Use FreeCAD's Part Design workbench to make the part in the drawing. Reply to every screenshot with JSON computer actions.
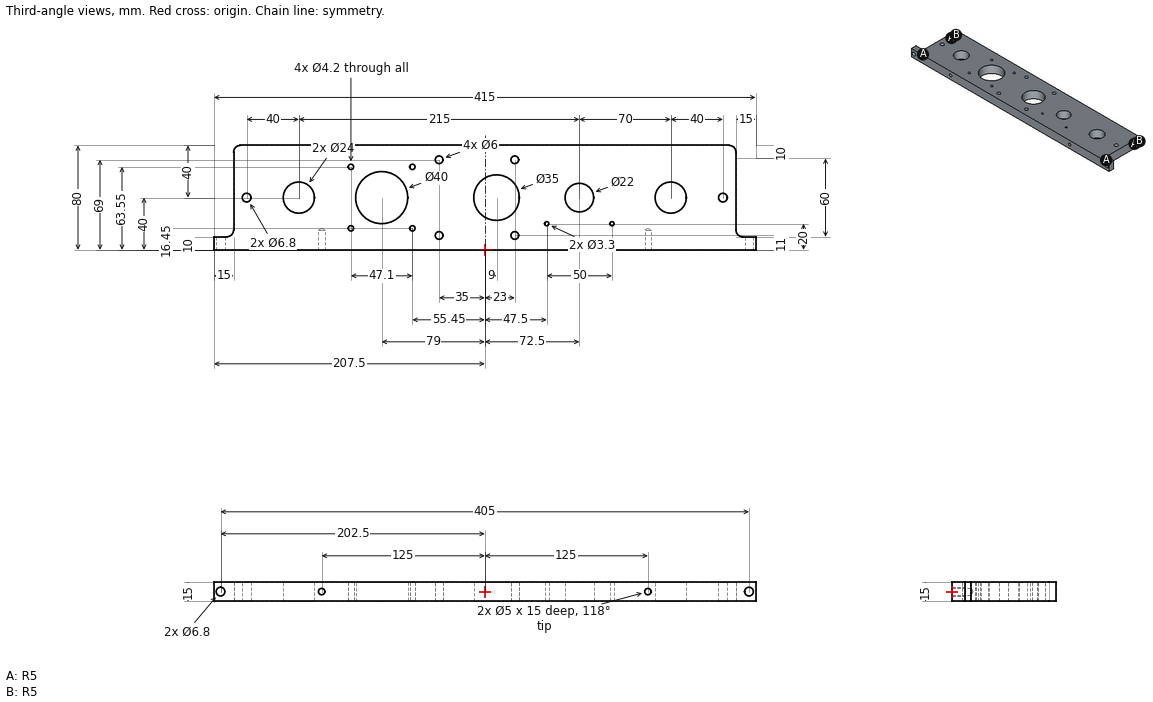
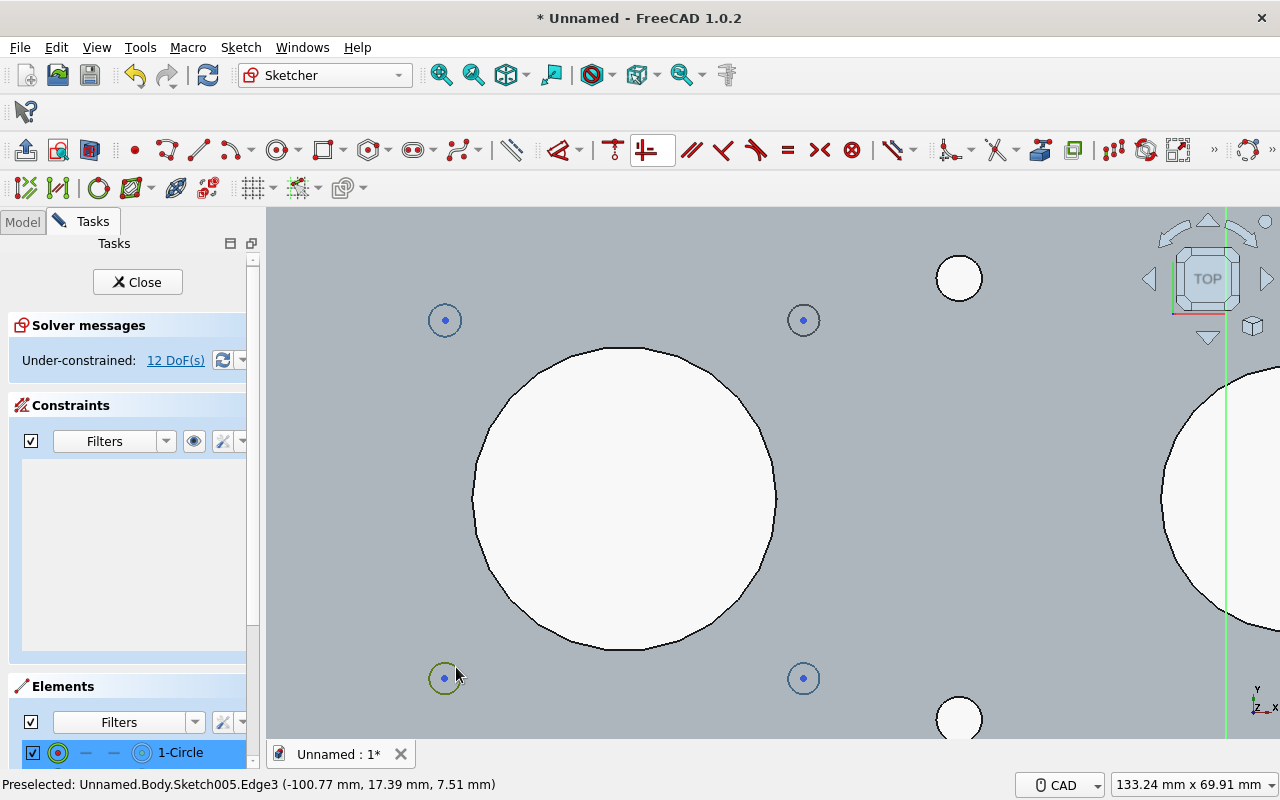
{"action": "left_click", "coordinate": [815, 309]}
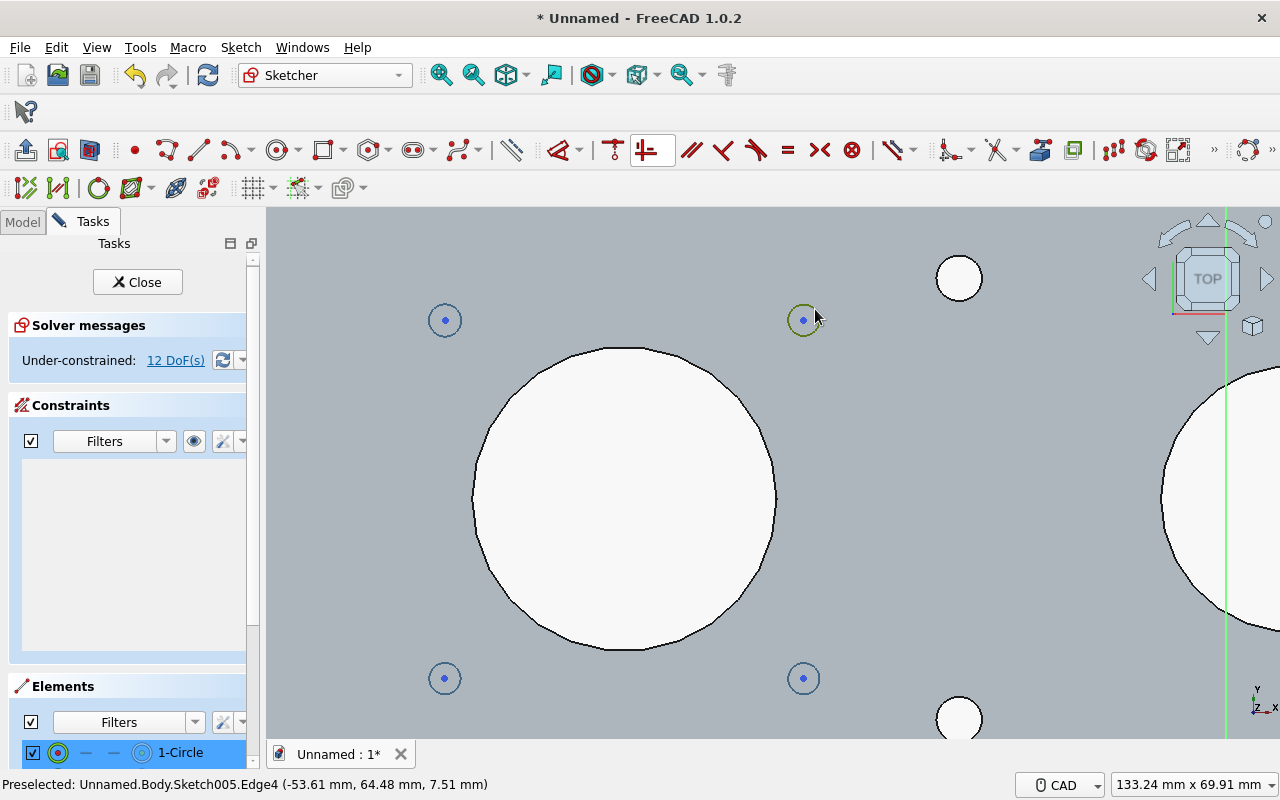
{"action": "left_click", "coordinate": [788, 150]}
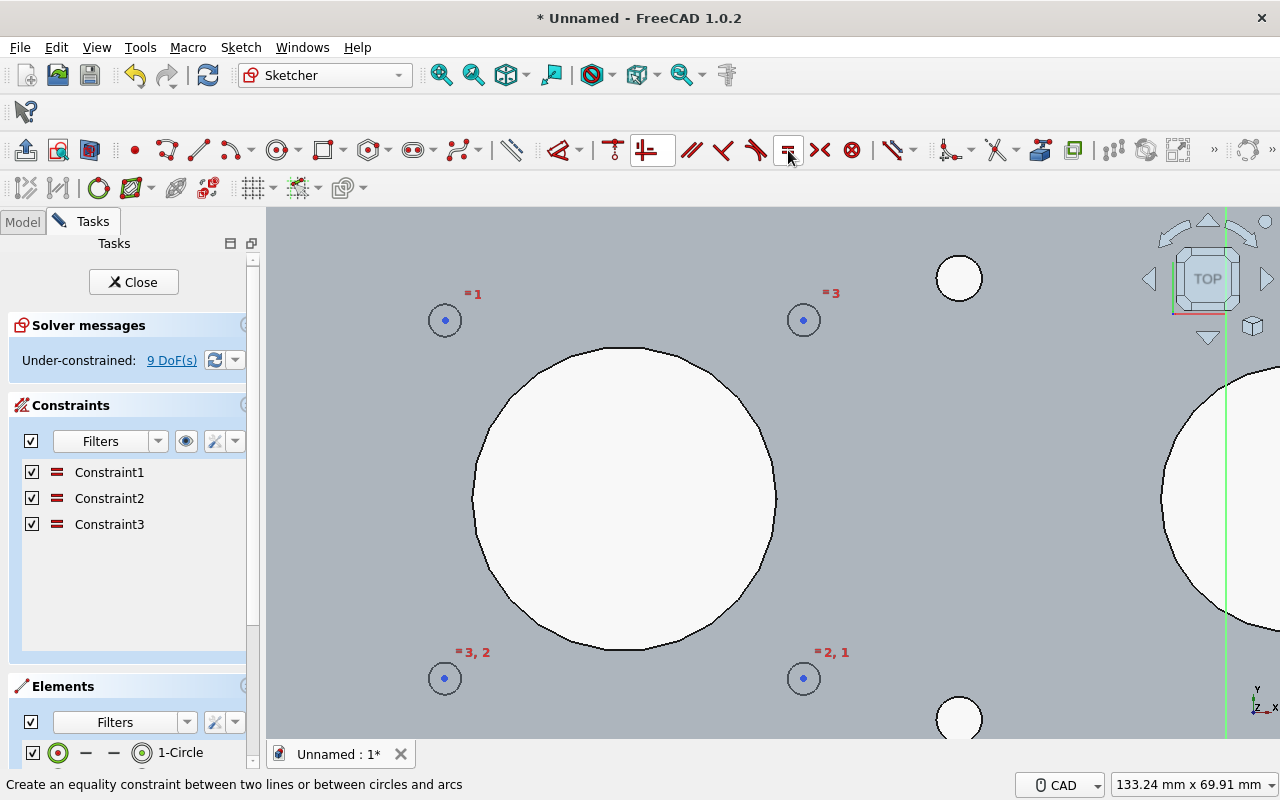
{"action": "left_click", "coordinate": [445, 320]}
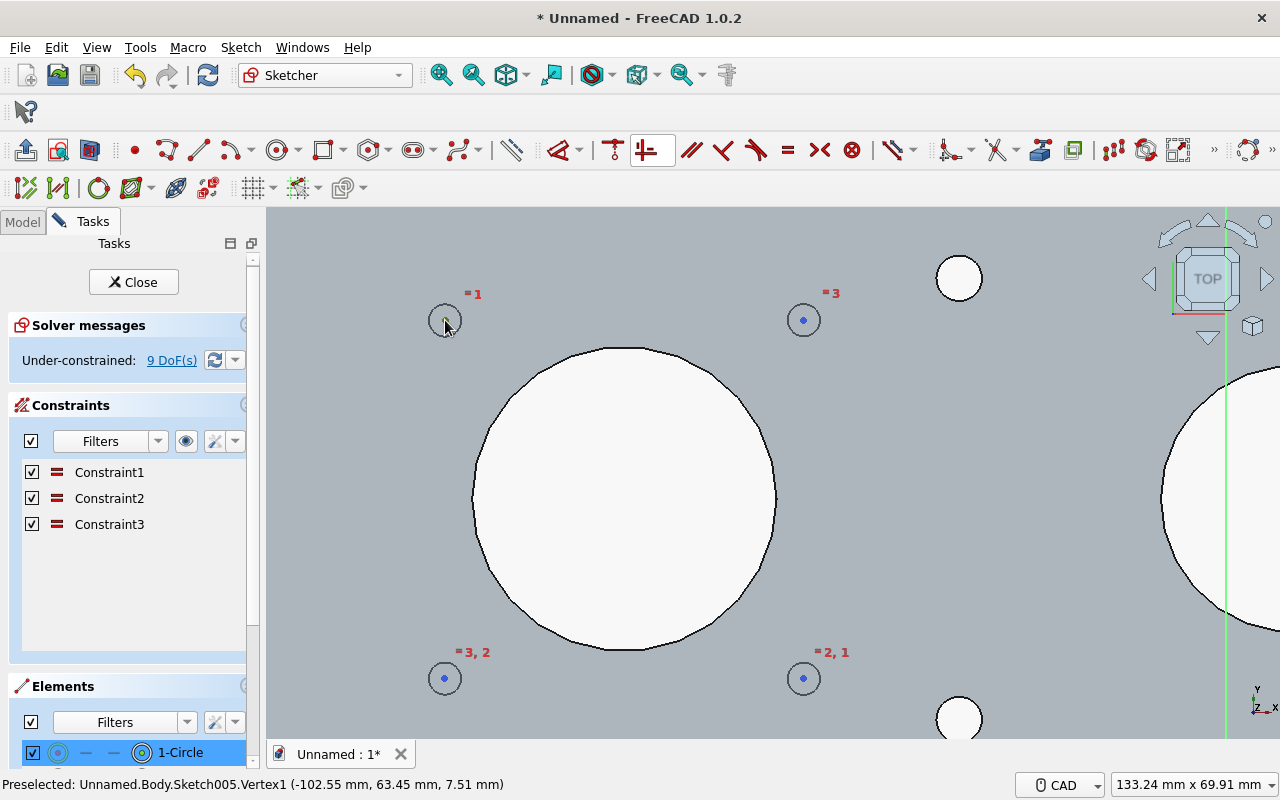
{"action": "left_click", "coordinate": [445, 679]}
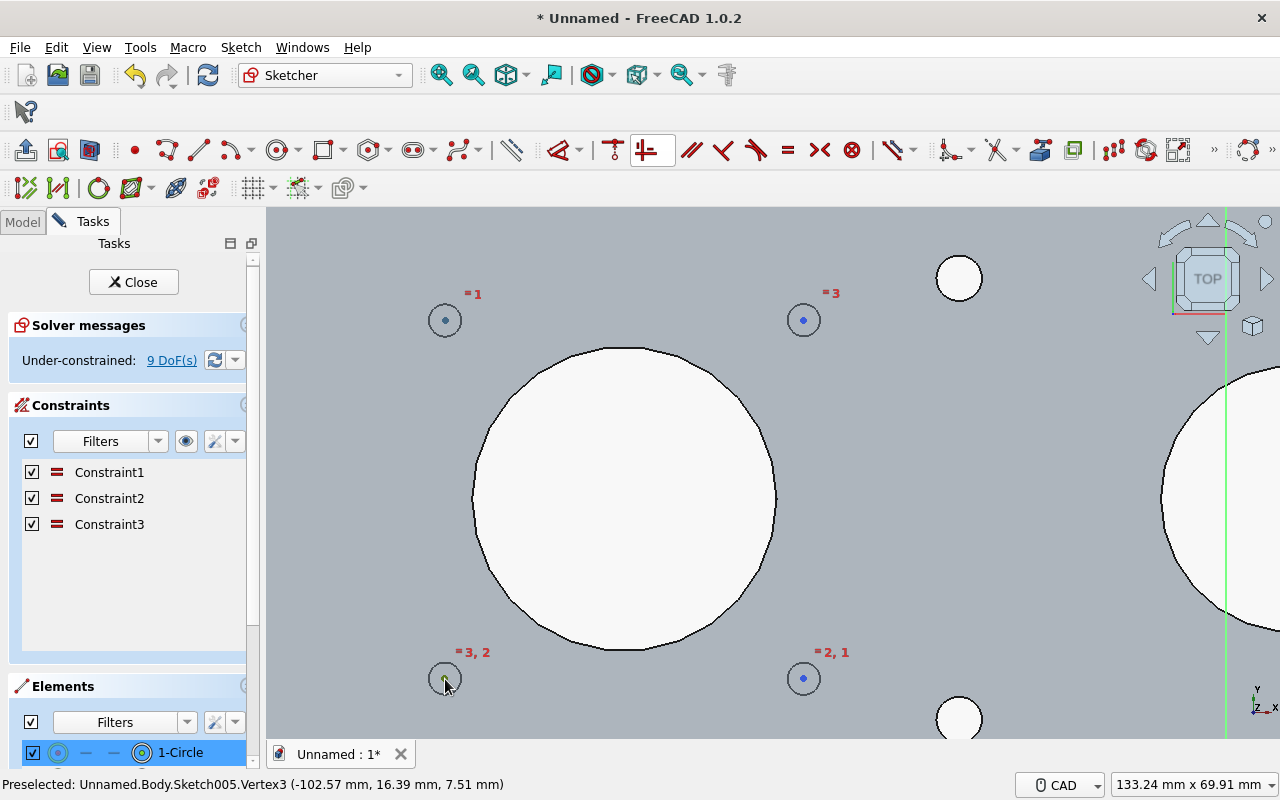
{"action": "key", "text": "v"}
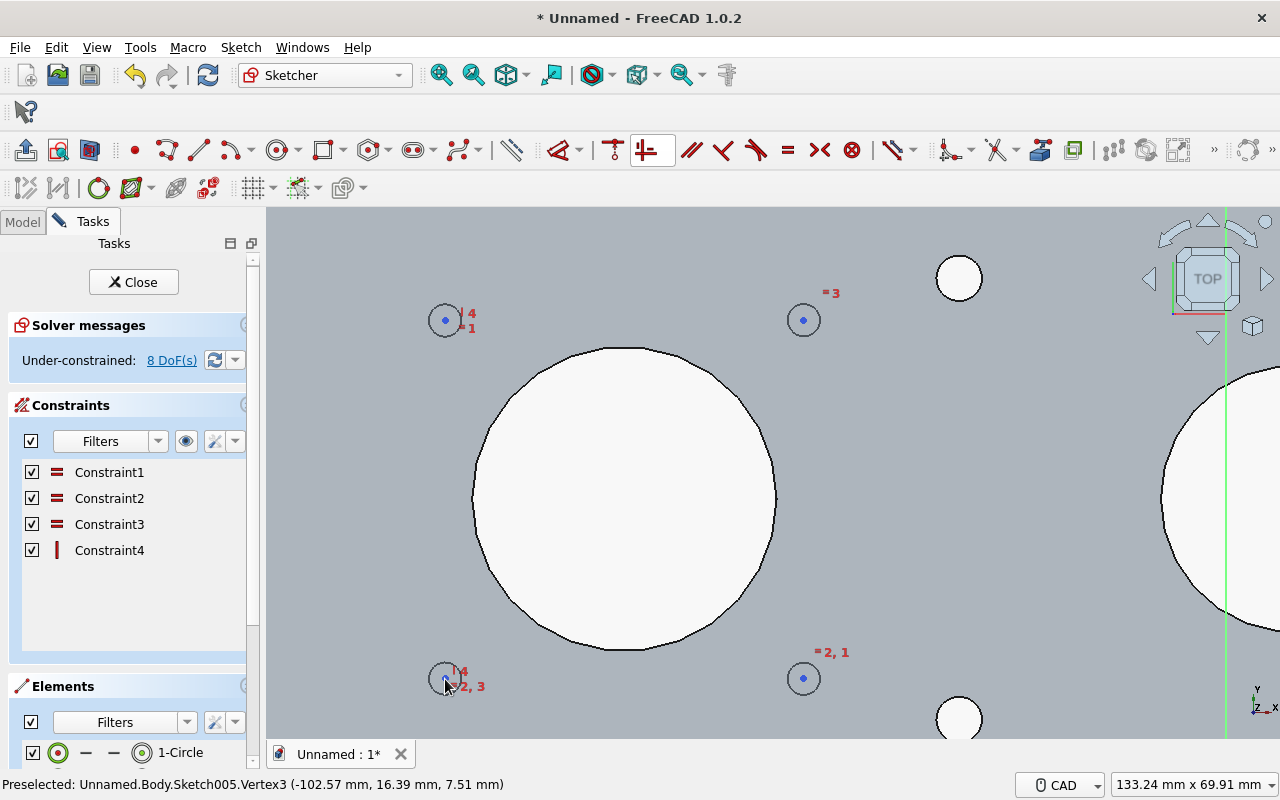
{"action": "left_click", "coordinate": [804, 679]}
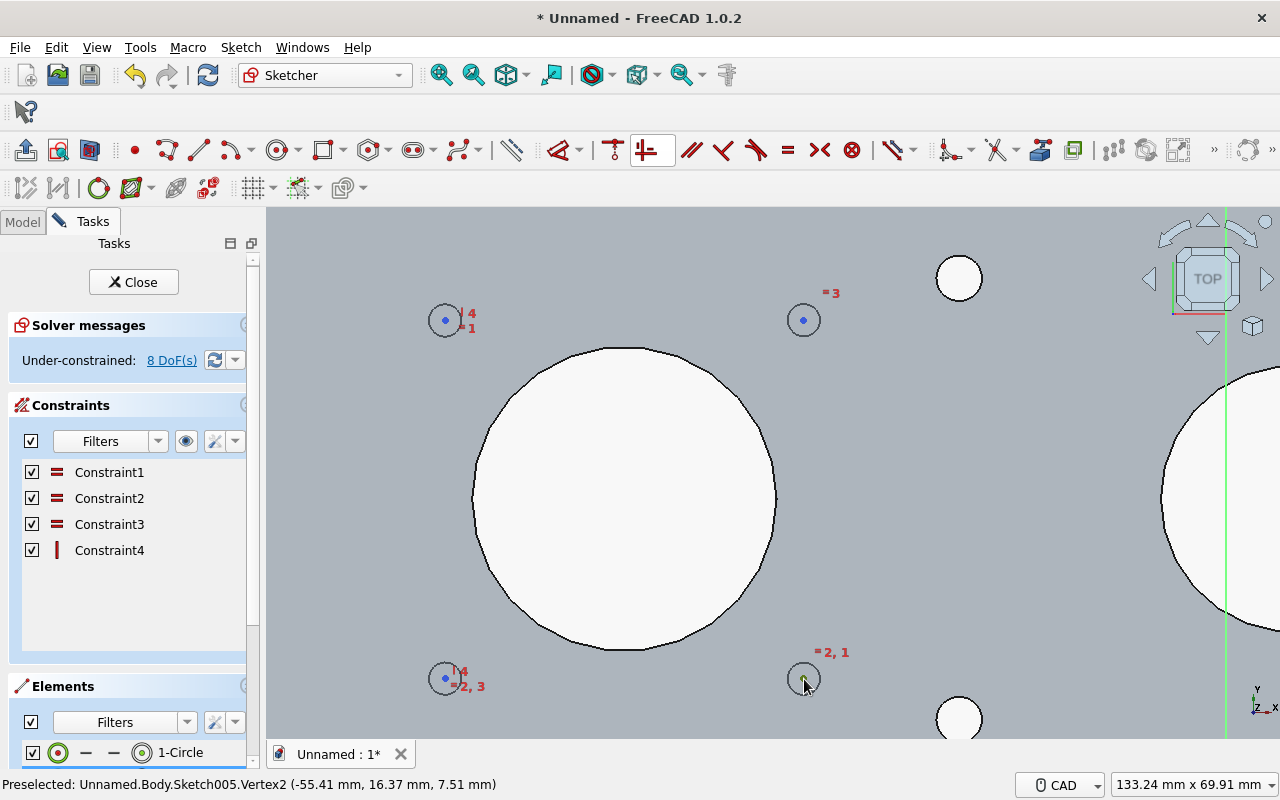
{"action": "left_click", "coordinate": [445, 679]}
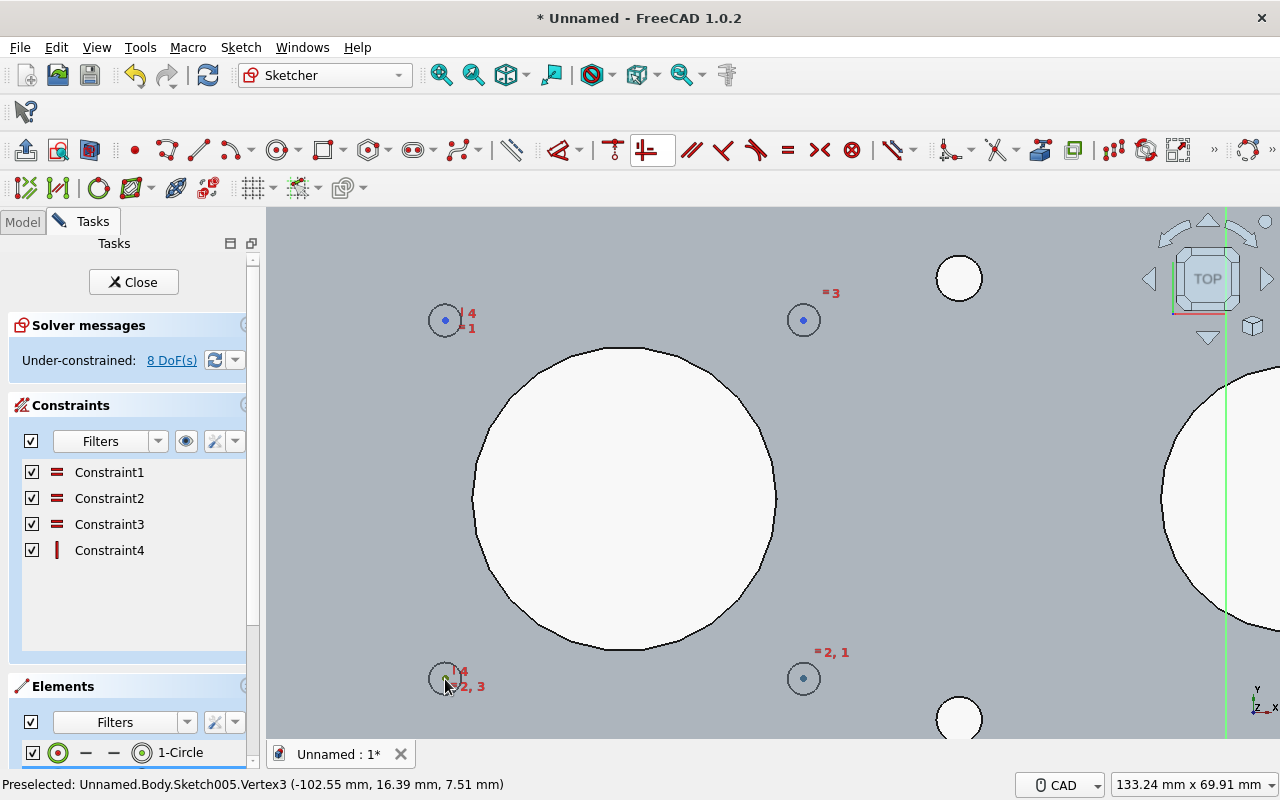
{"action": "left_click", "coordinate": [670, 150]}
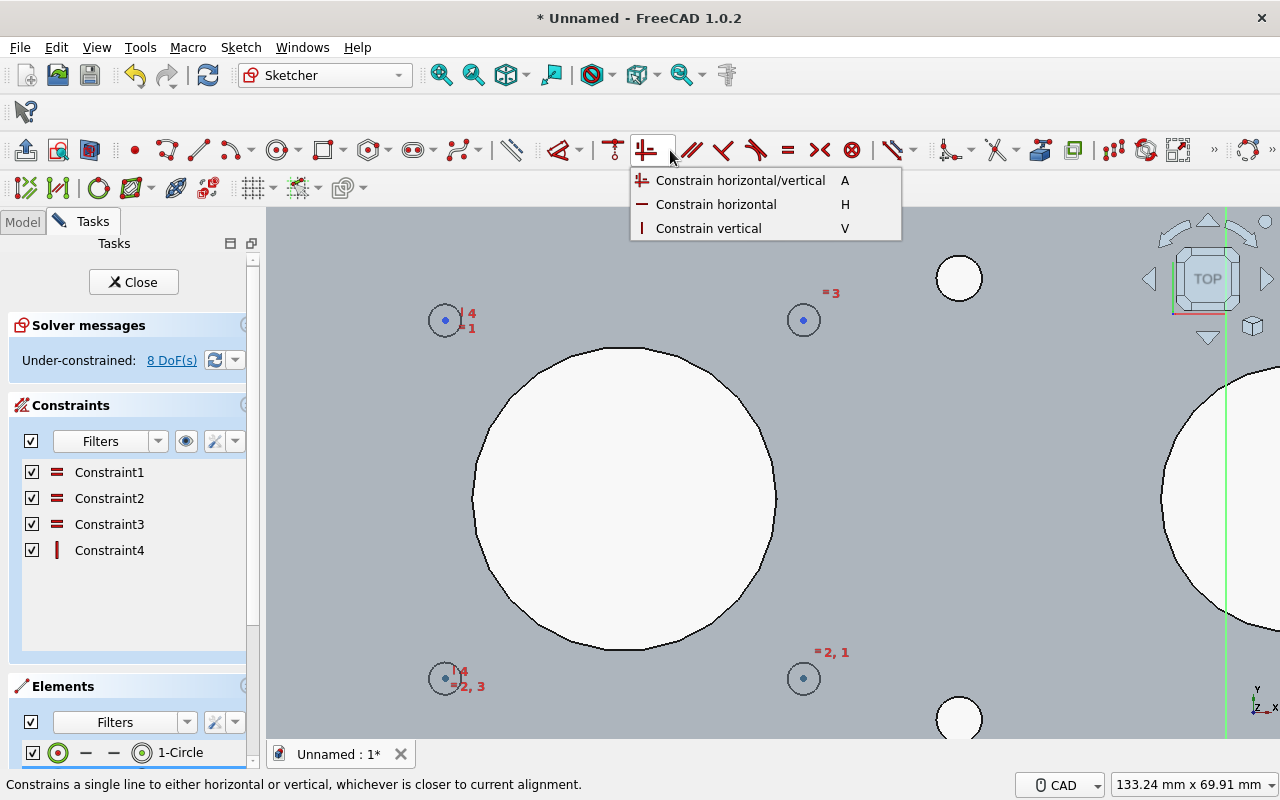
{"action": "left_click", "coordinate": [766, 204]}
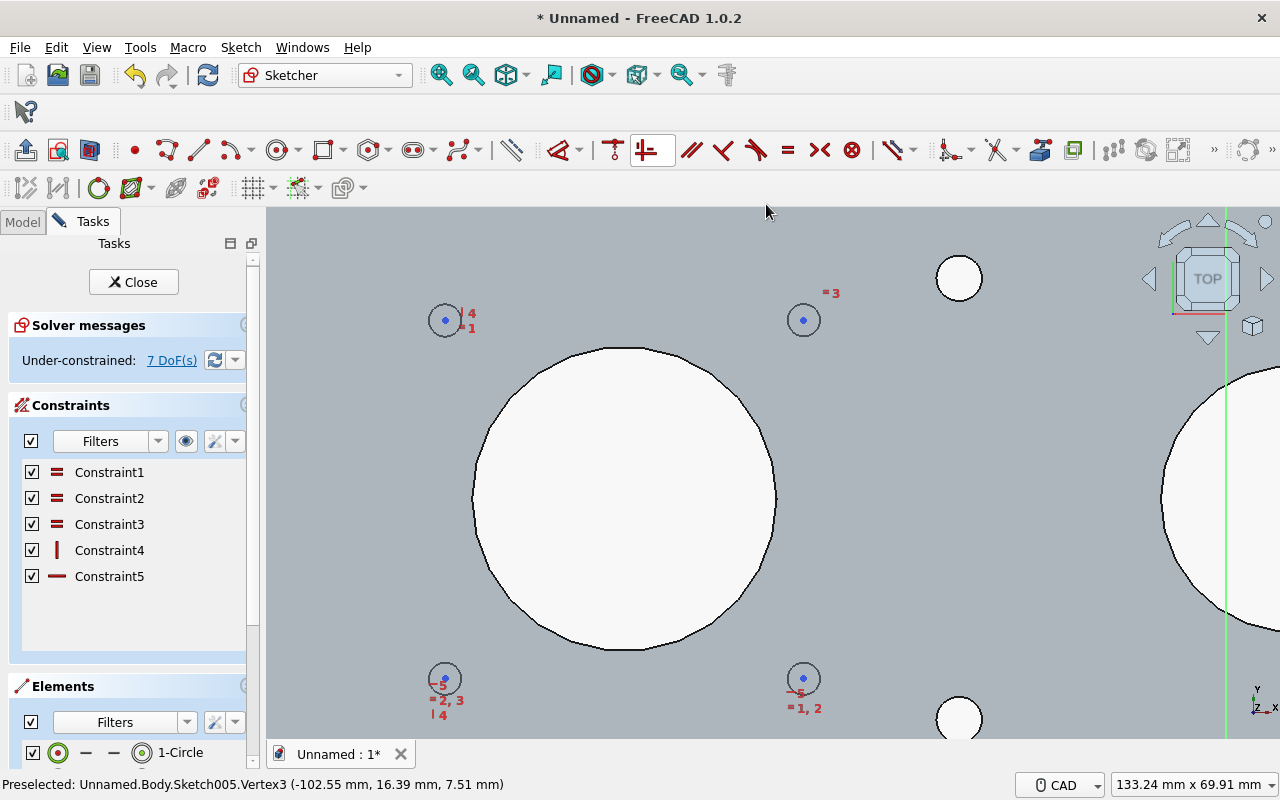
{"action": "left_click", "coordinate": [804, 679]}